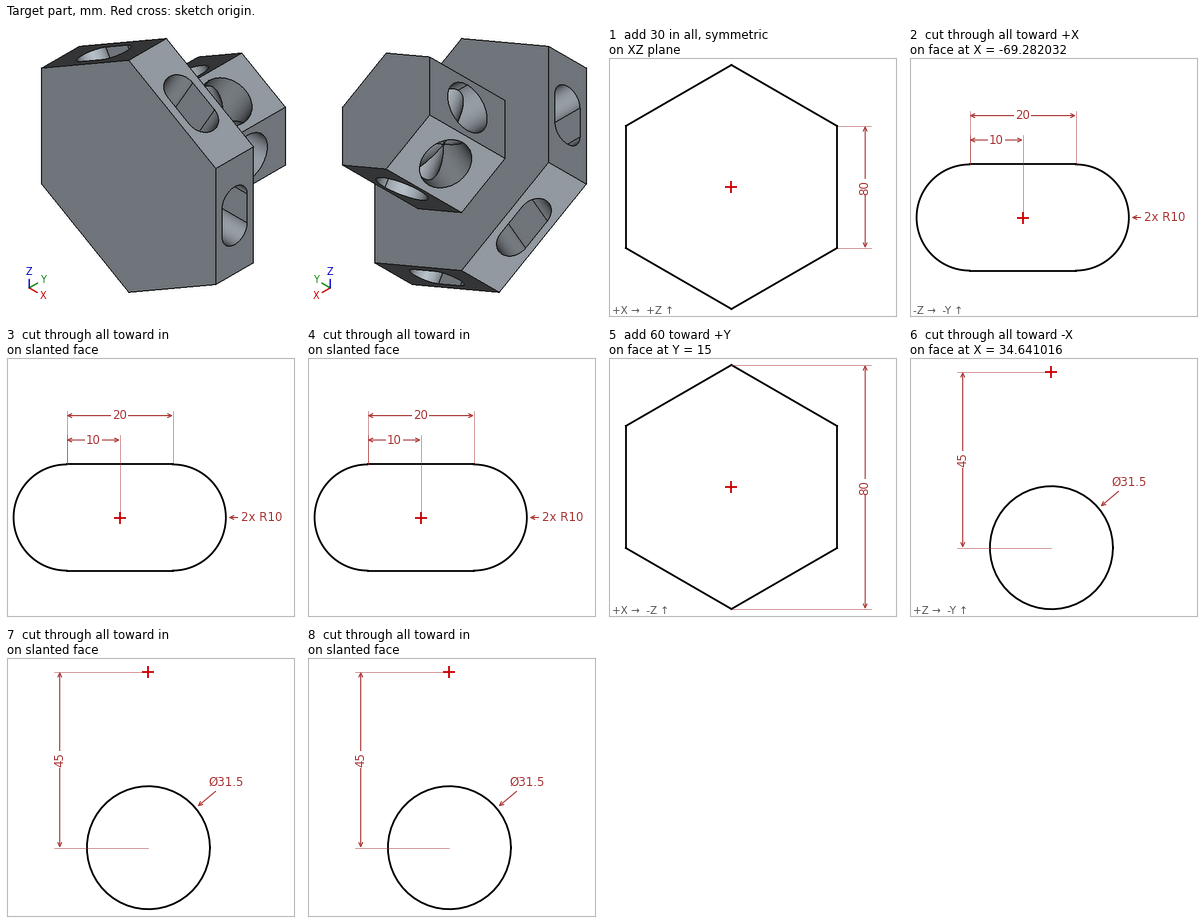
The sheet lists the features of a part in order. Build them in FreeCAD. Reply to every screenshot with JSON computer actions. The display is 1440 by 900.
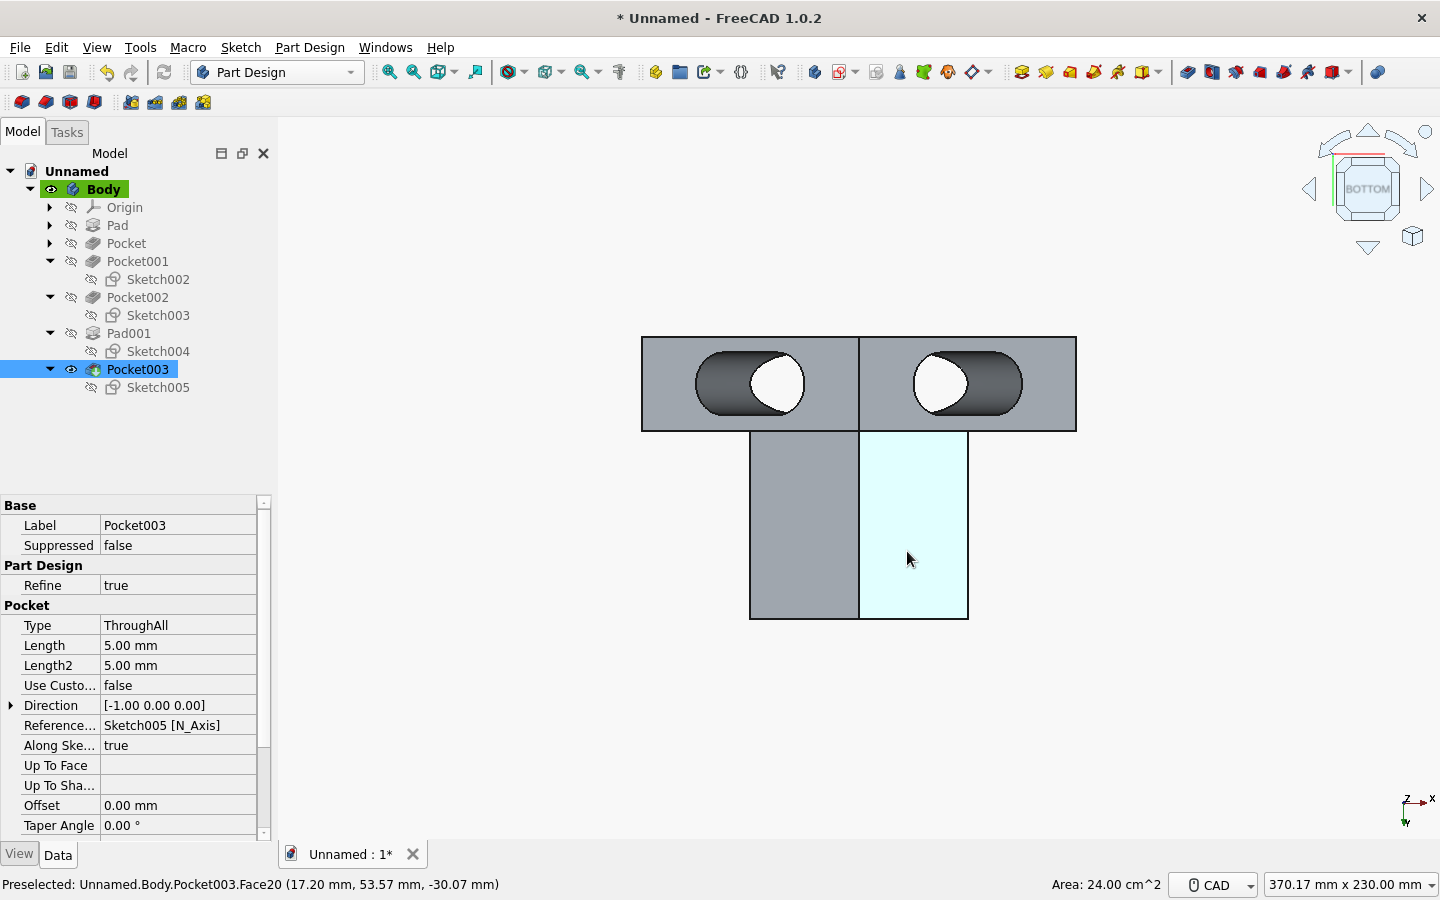
{"action": "left_click", "coordinate": [840, 72]}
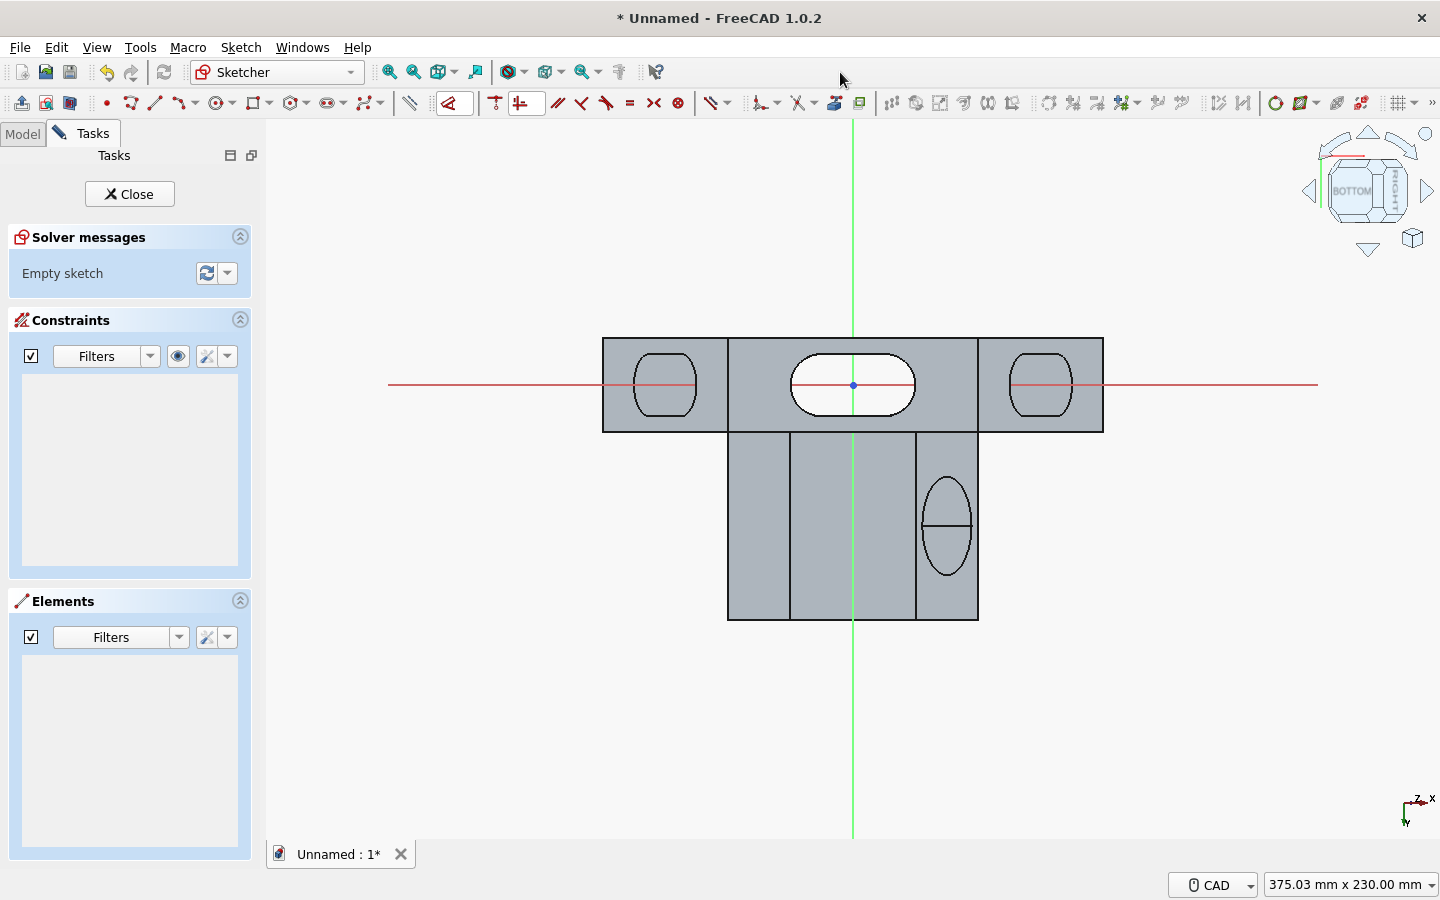
{"action": "left_click", "coordinate": [70, 104]}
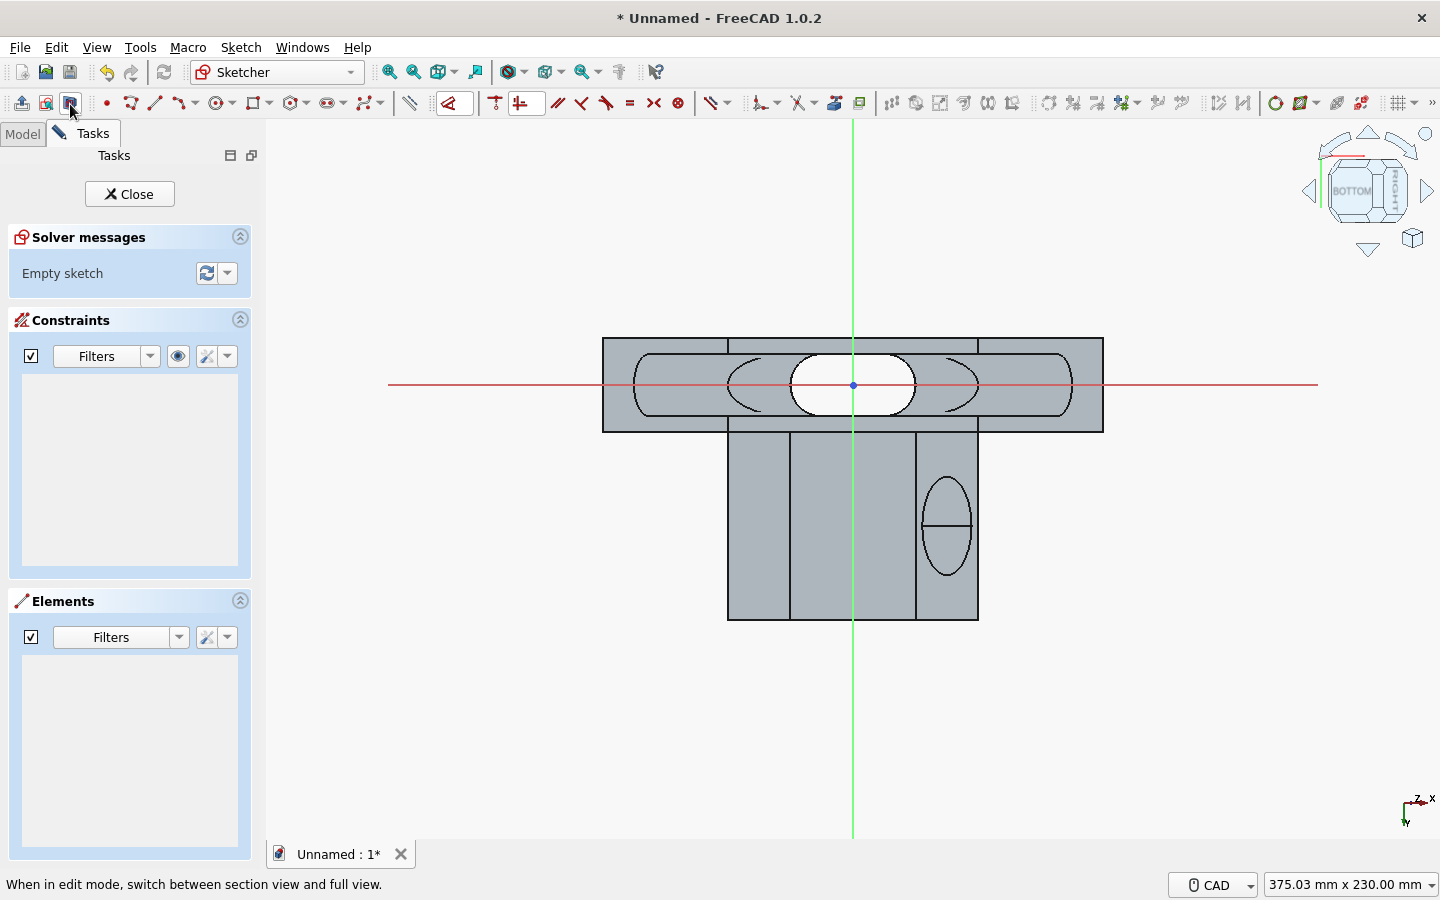
{"action": "scroll", "coordinate": [893, 481], "scroll_direction": "up", "scroll_amount": 5}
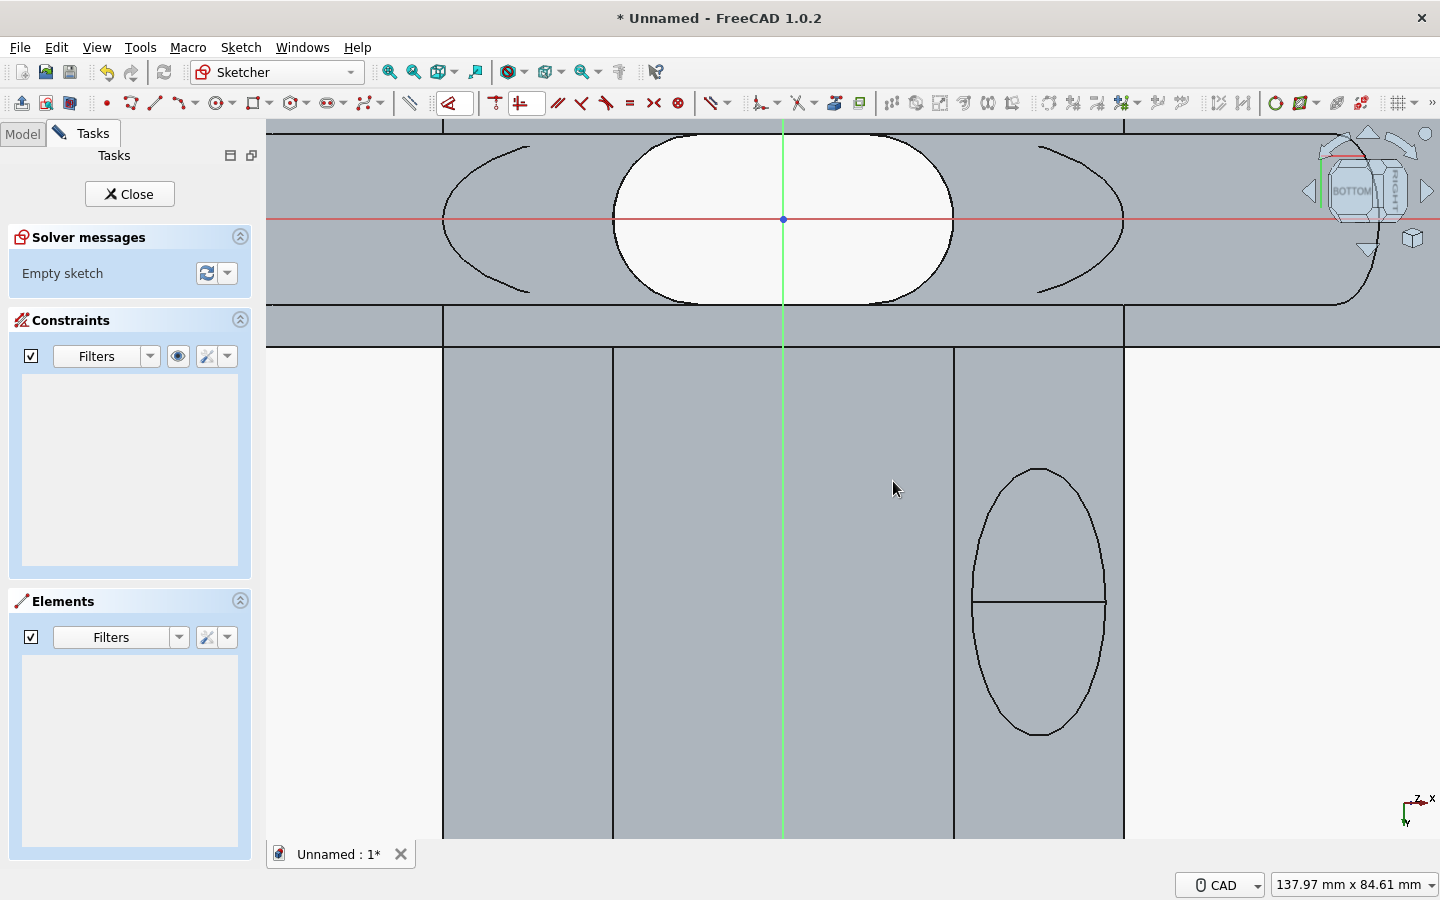
{"action": "left_click", "coordinate": [216, 104]}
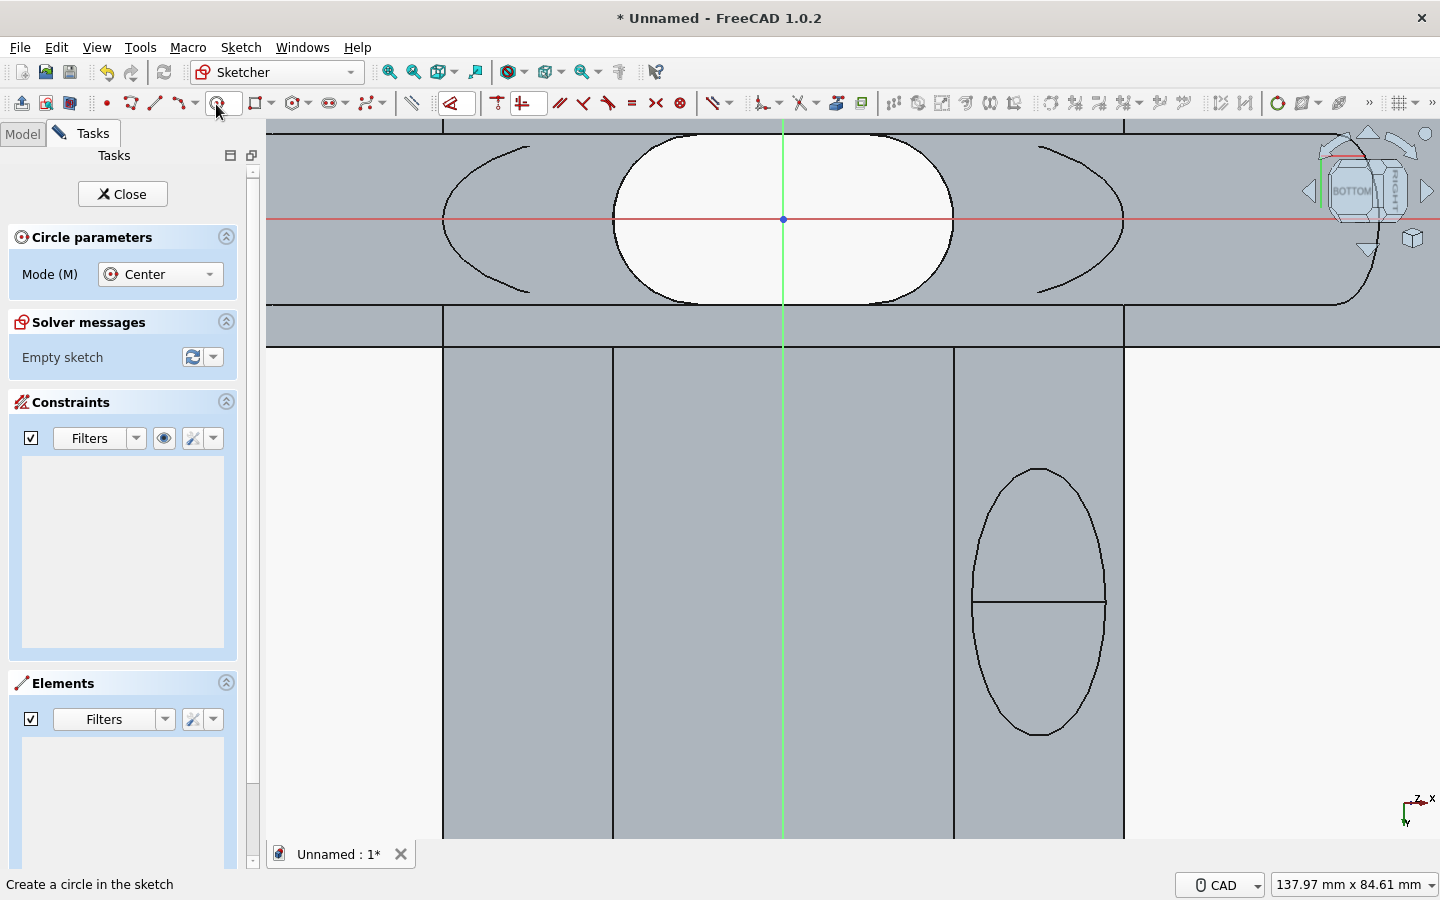
{"action": "left_click", "coordinate": [783, 602]}
{"action": "mouse_move", "coordinate": [878, 508]}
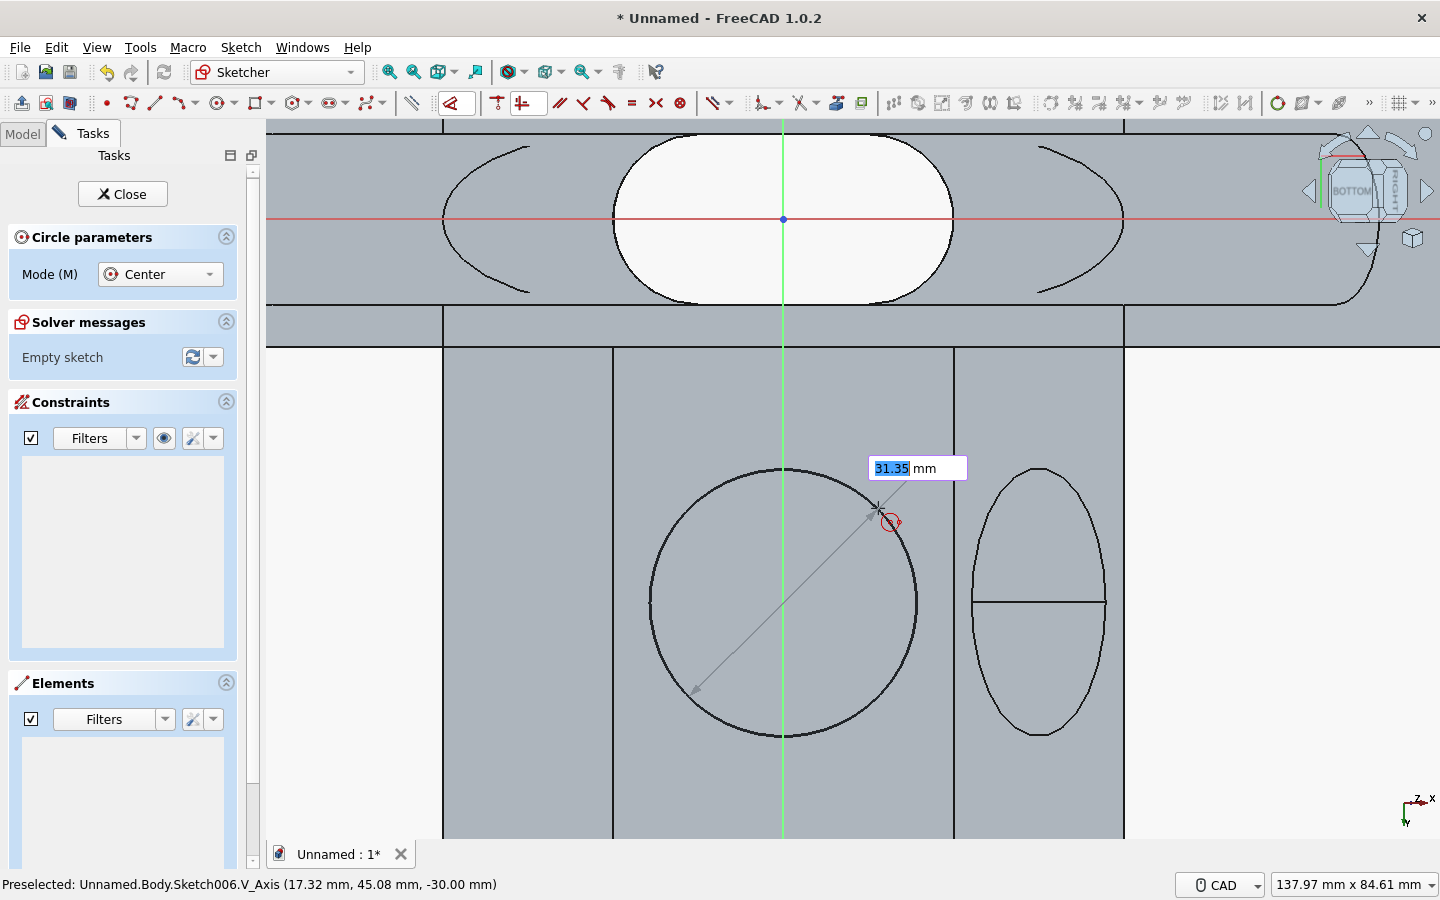
{"action": "type", "text": "31.5"}
{"action": "key", "text": "Return"}
{"action": "key", "text": "Escape"}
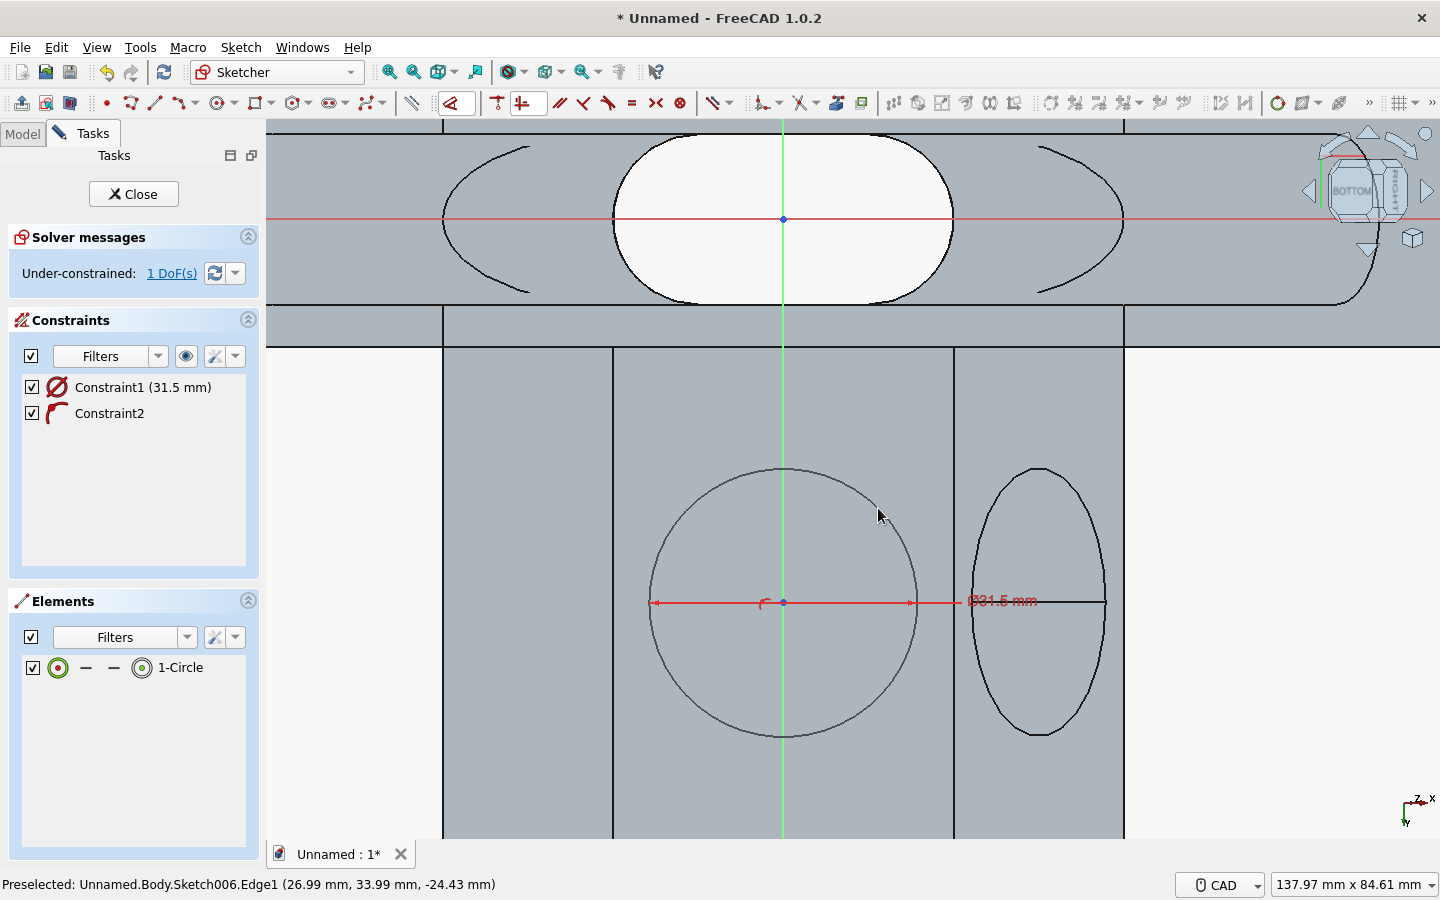
{"action": "left_click", "coordinate": [783, 603]}